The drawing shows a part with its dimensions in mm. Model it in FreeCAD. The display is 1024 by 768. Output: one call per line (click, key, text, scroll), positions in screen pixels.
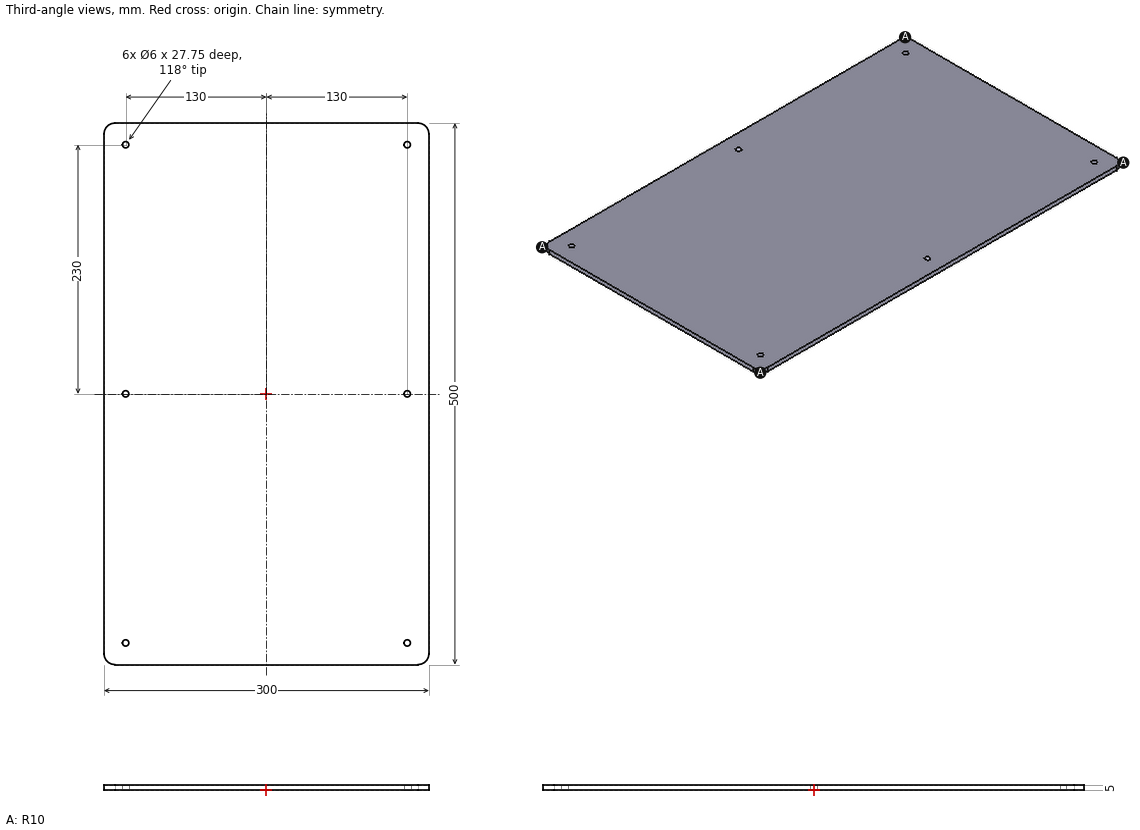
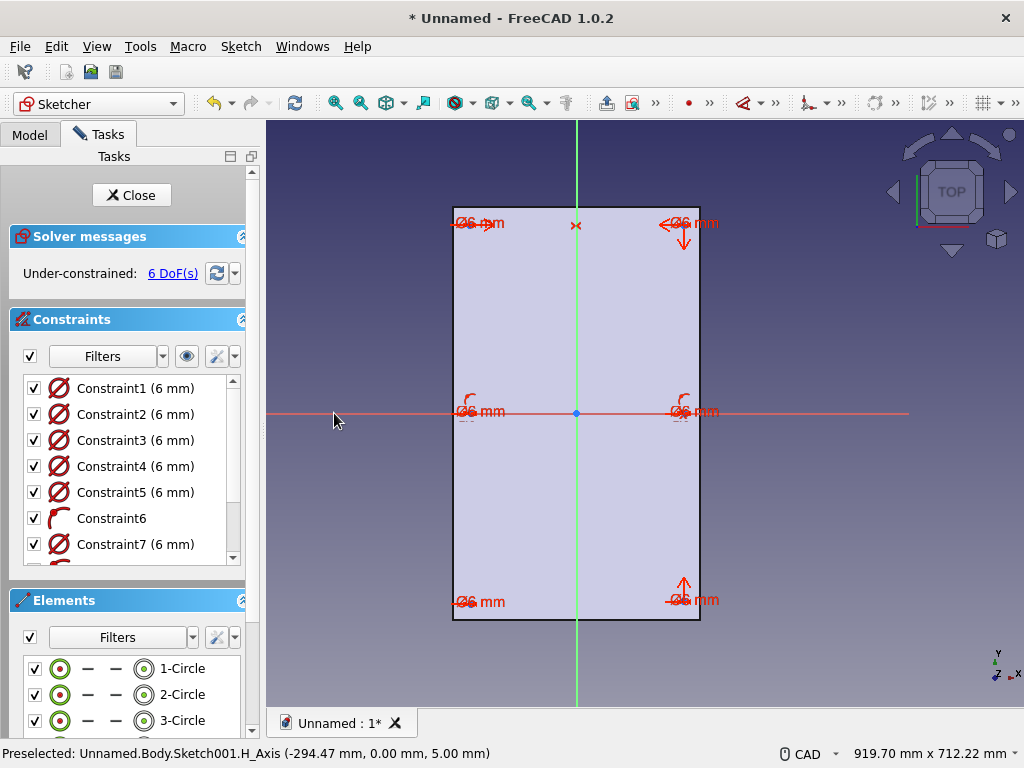
click(469, 225)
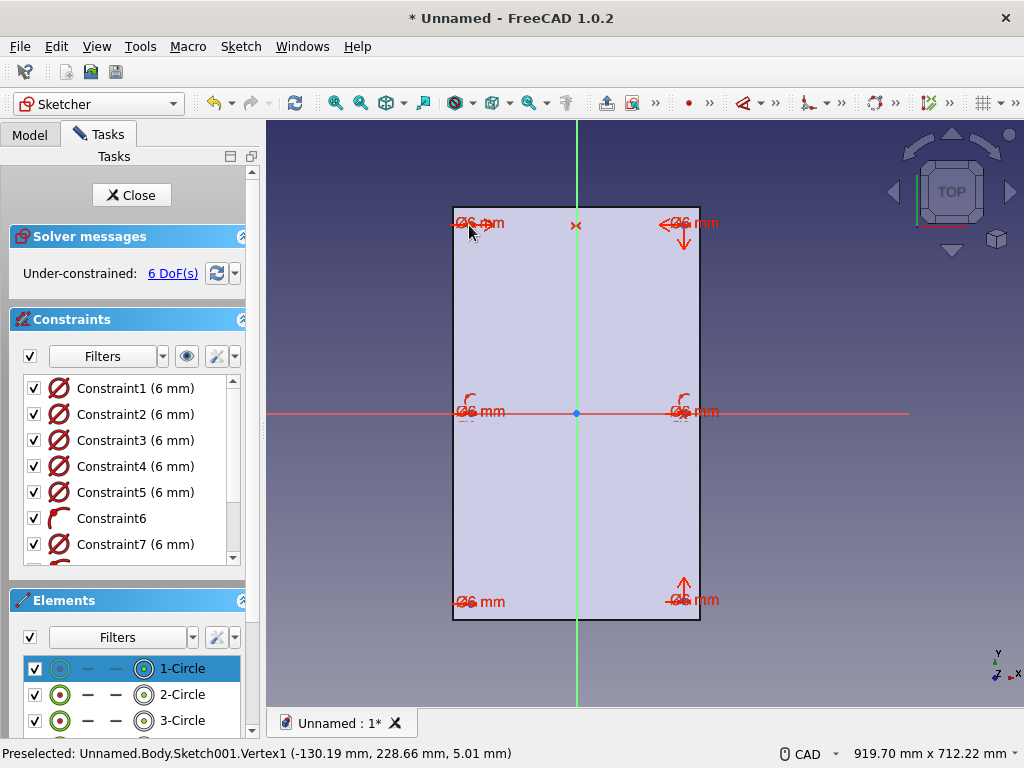
click(470, 604)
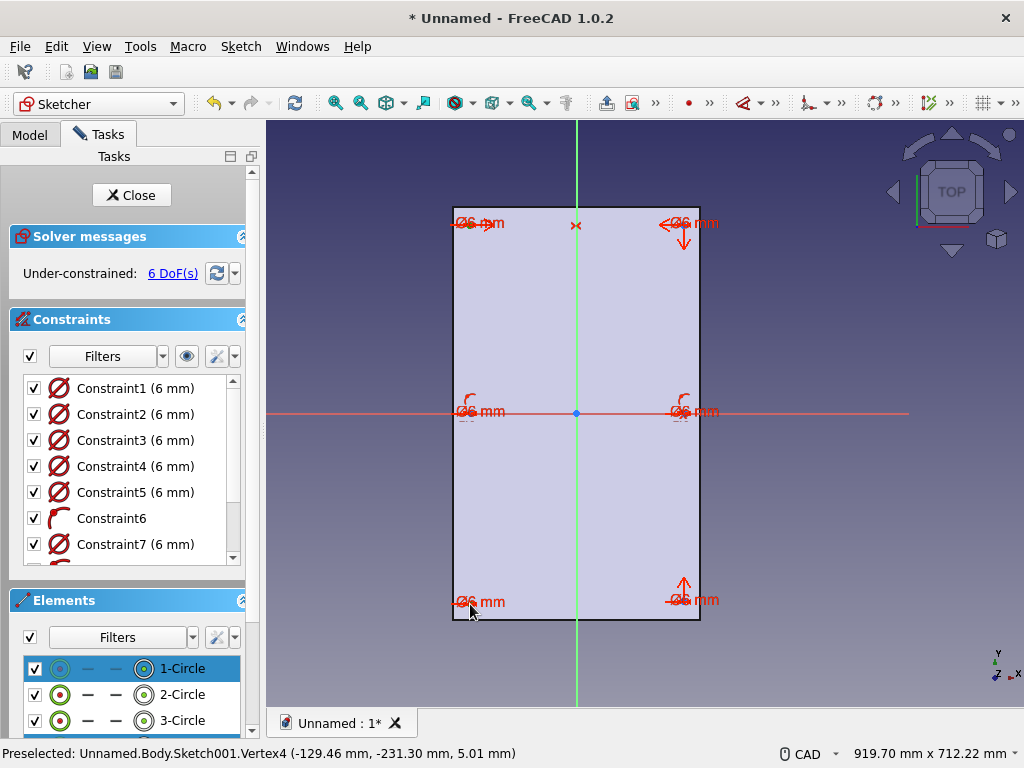
click(334, 413)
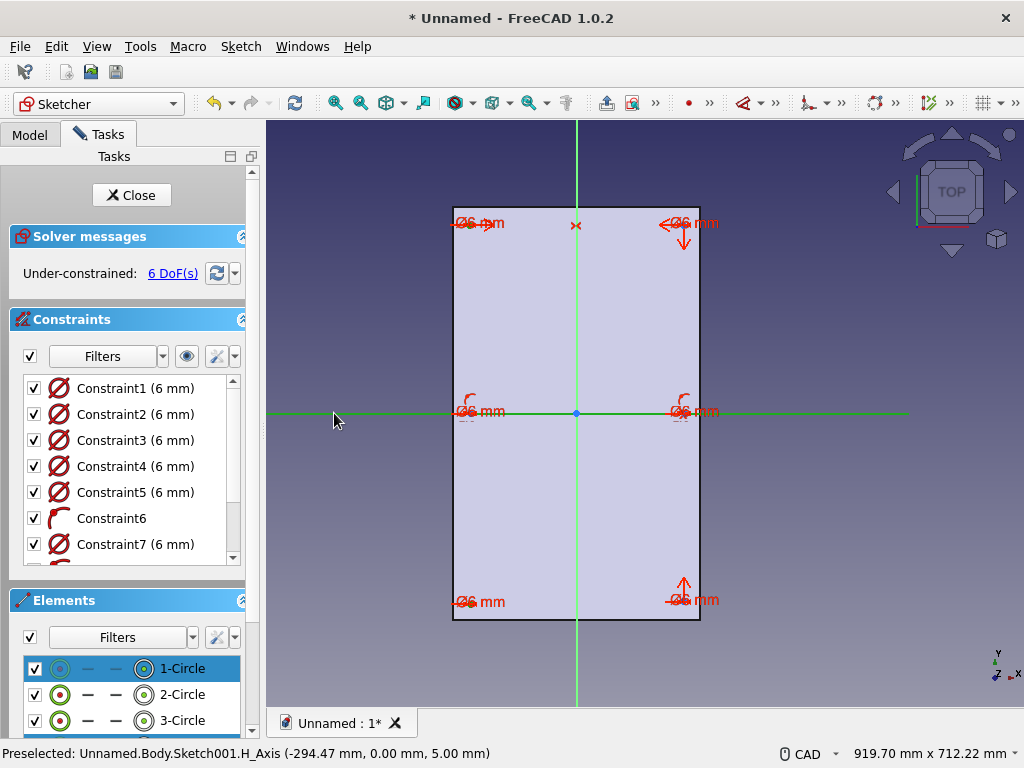
key(s)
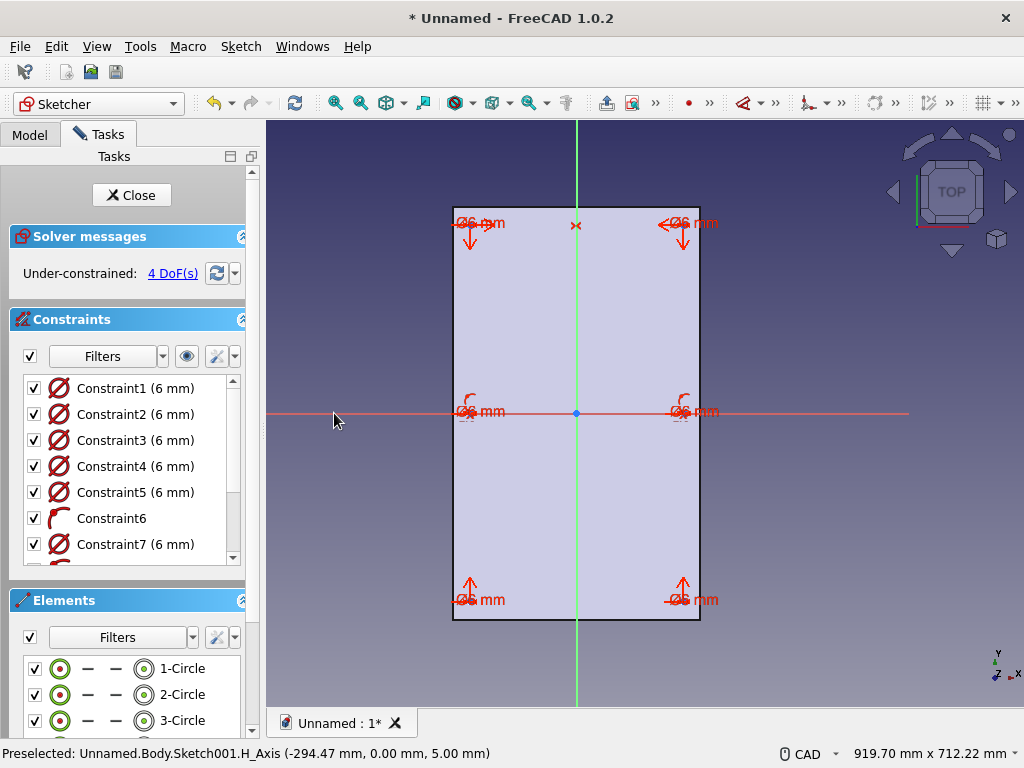
click(742, 104)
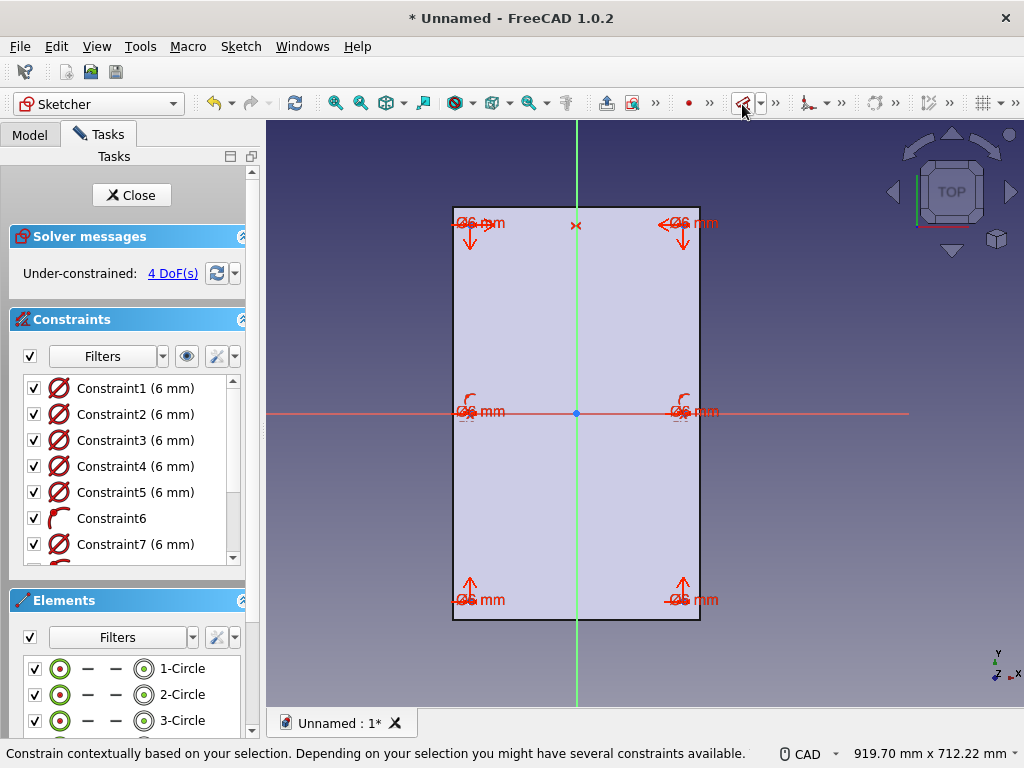
click(470, 225)
click(523, 191)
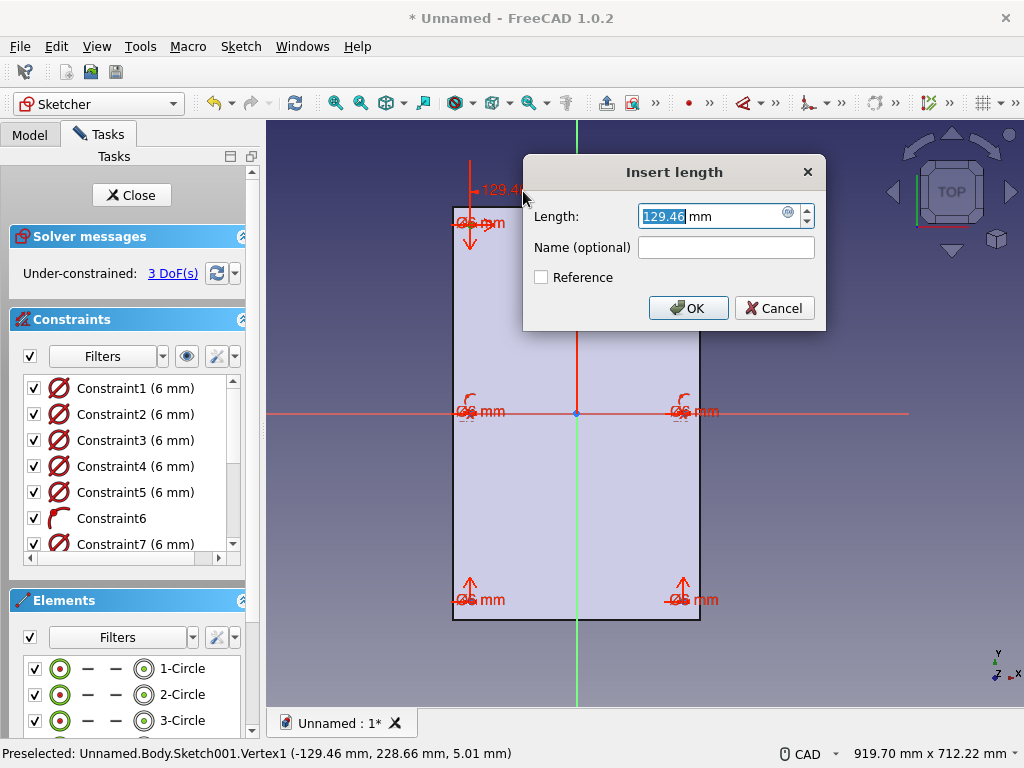
text(130)
key(Return)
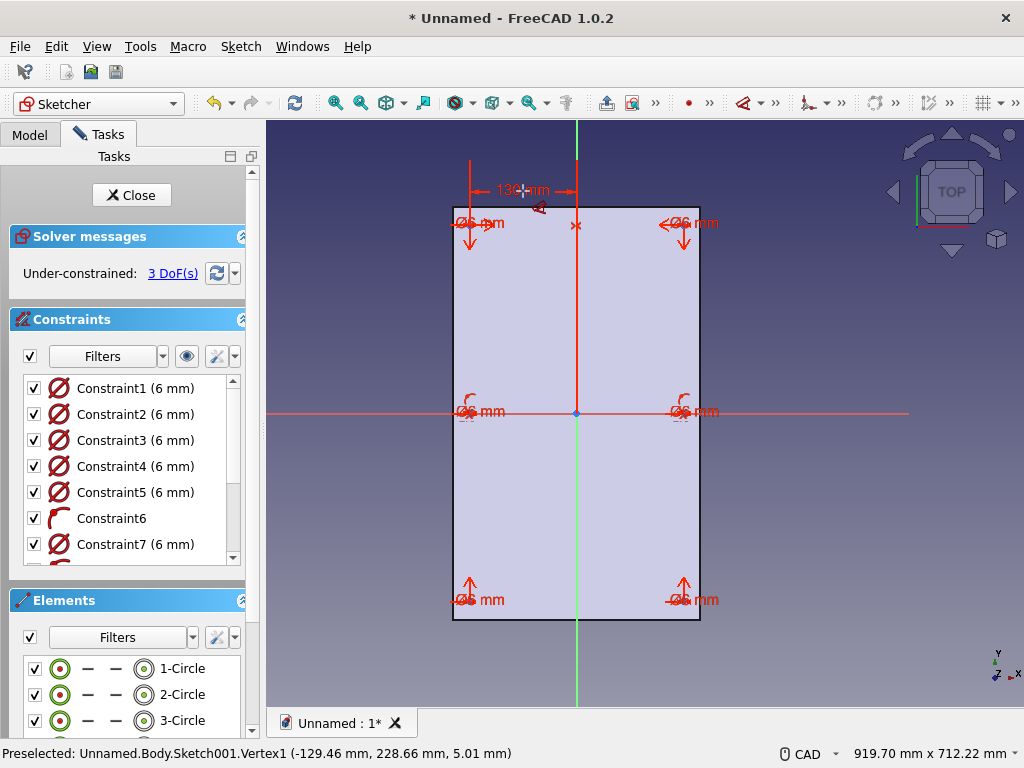
click(470, 225)
click(436, 319)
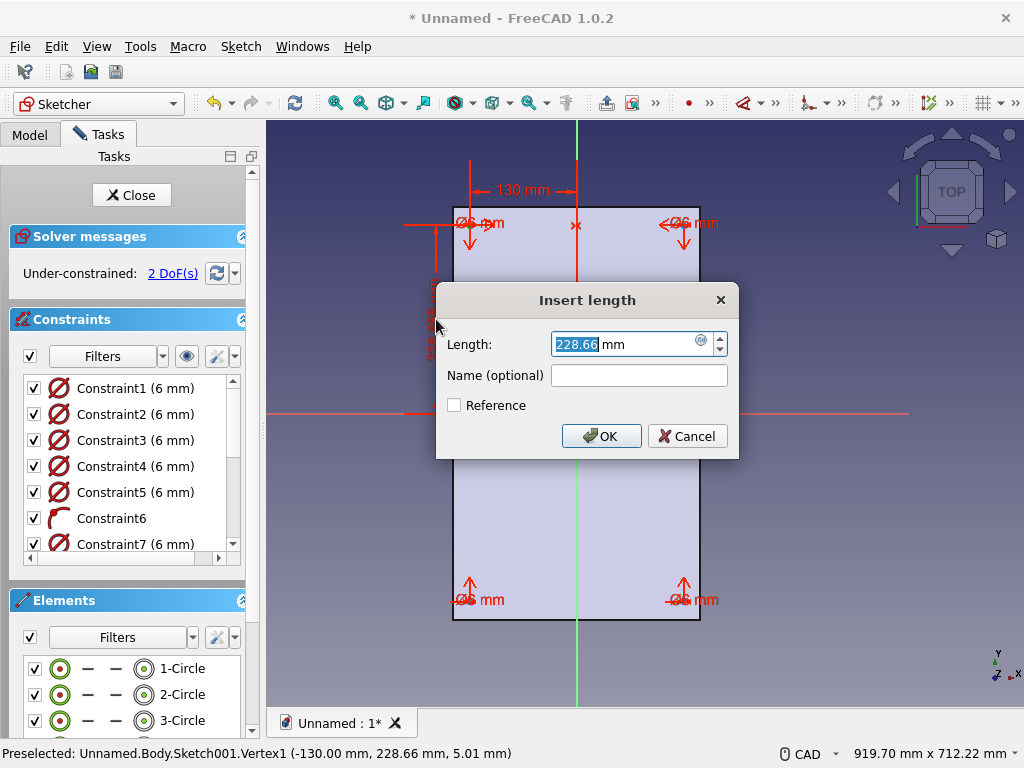
text(230)
key(Return)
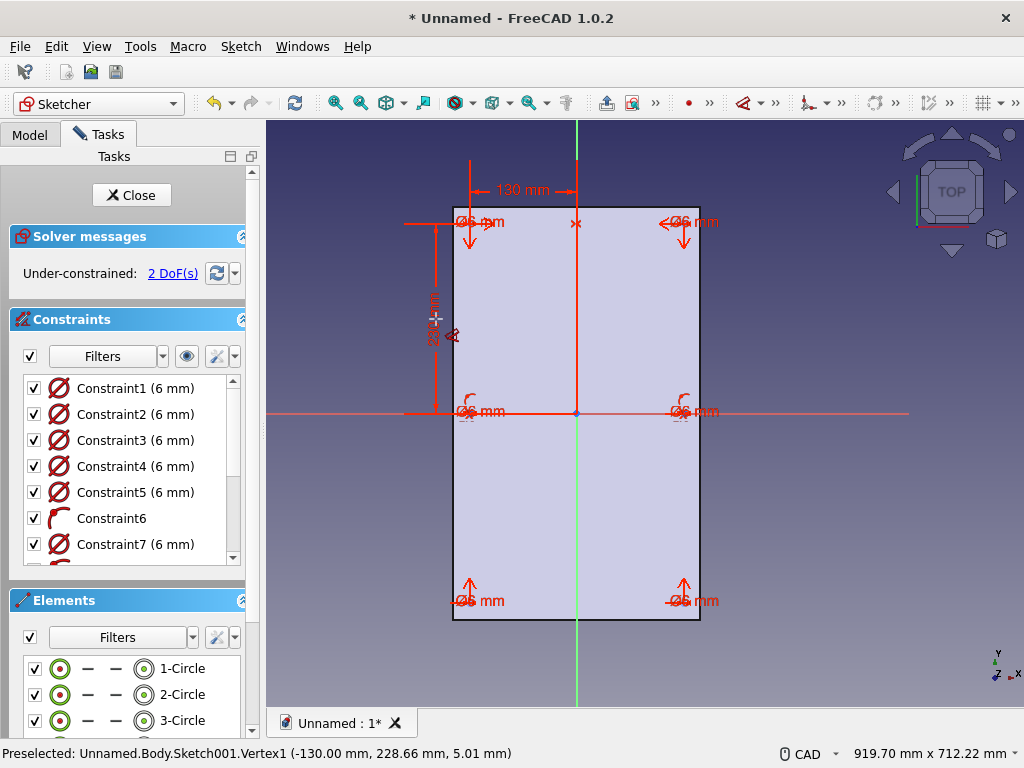
click(470, 413)
click(523, 447)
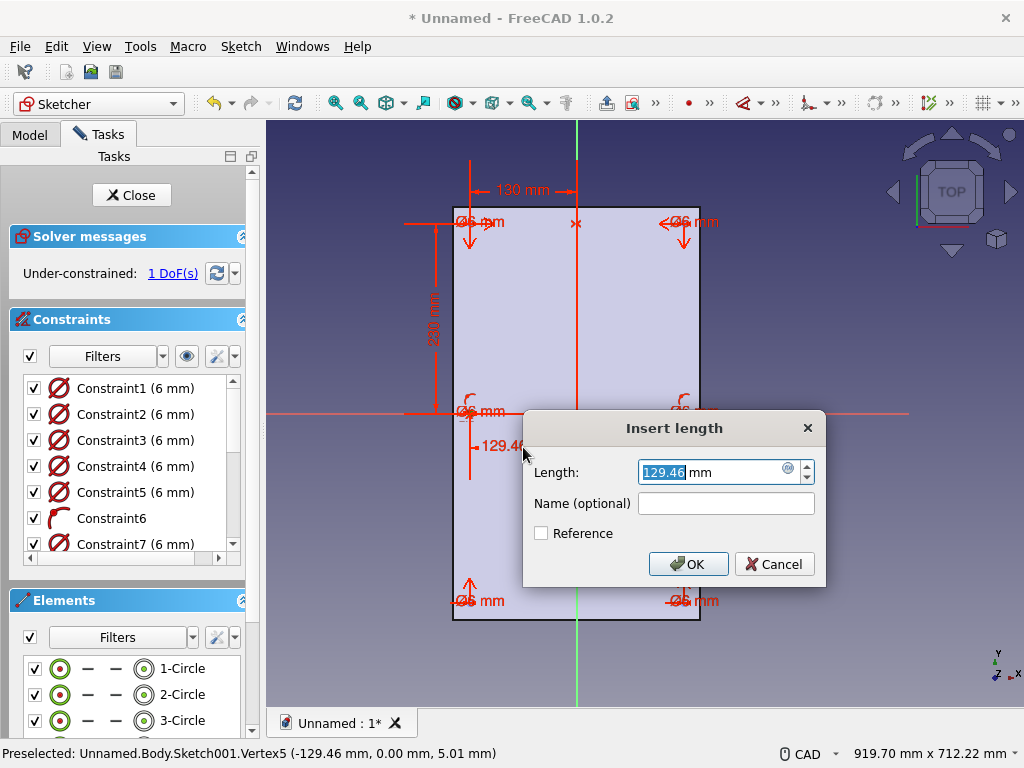
text(130)
key(Return)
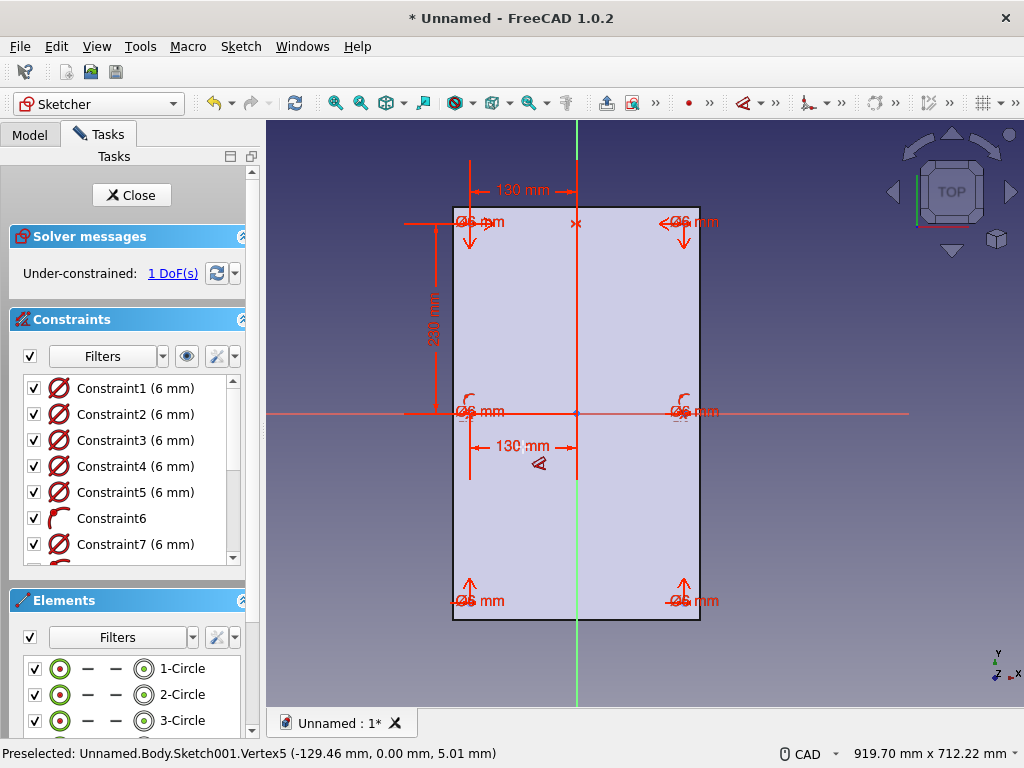
click(684, 413)
click(630, 447)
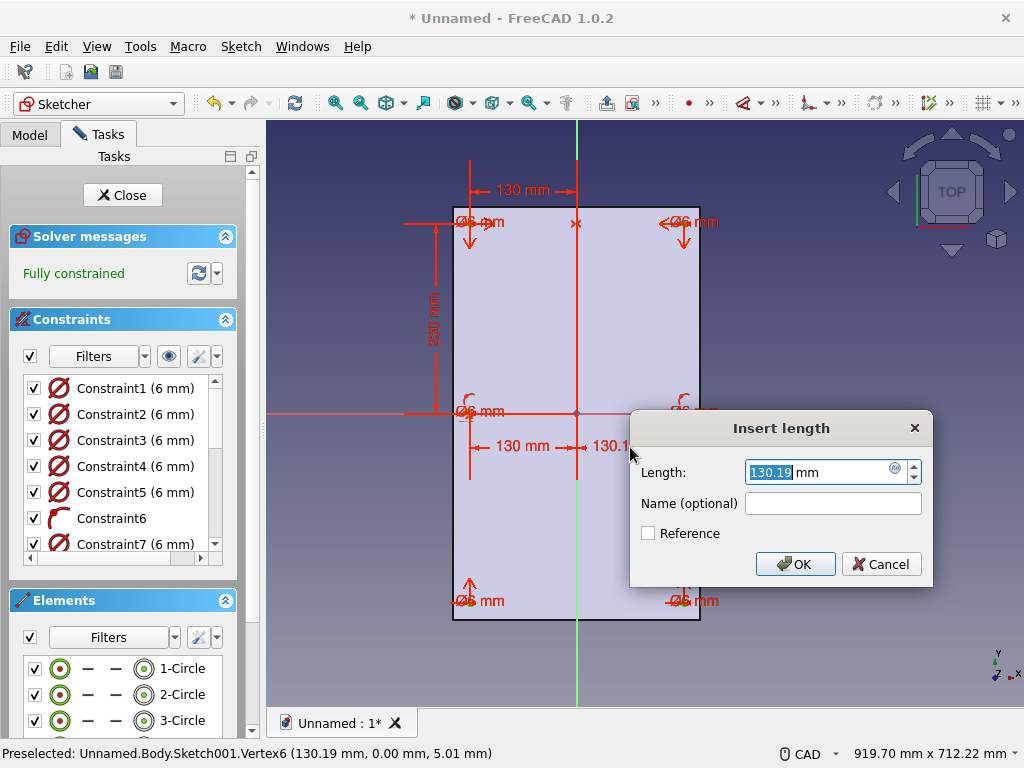
text(130)
key(Return)
key(Escape)